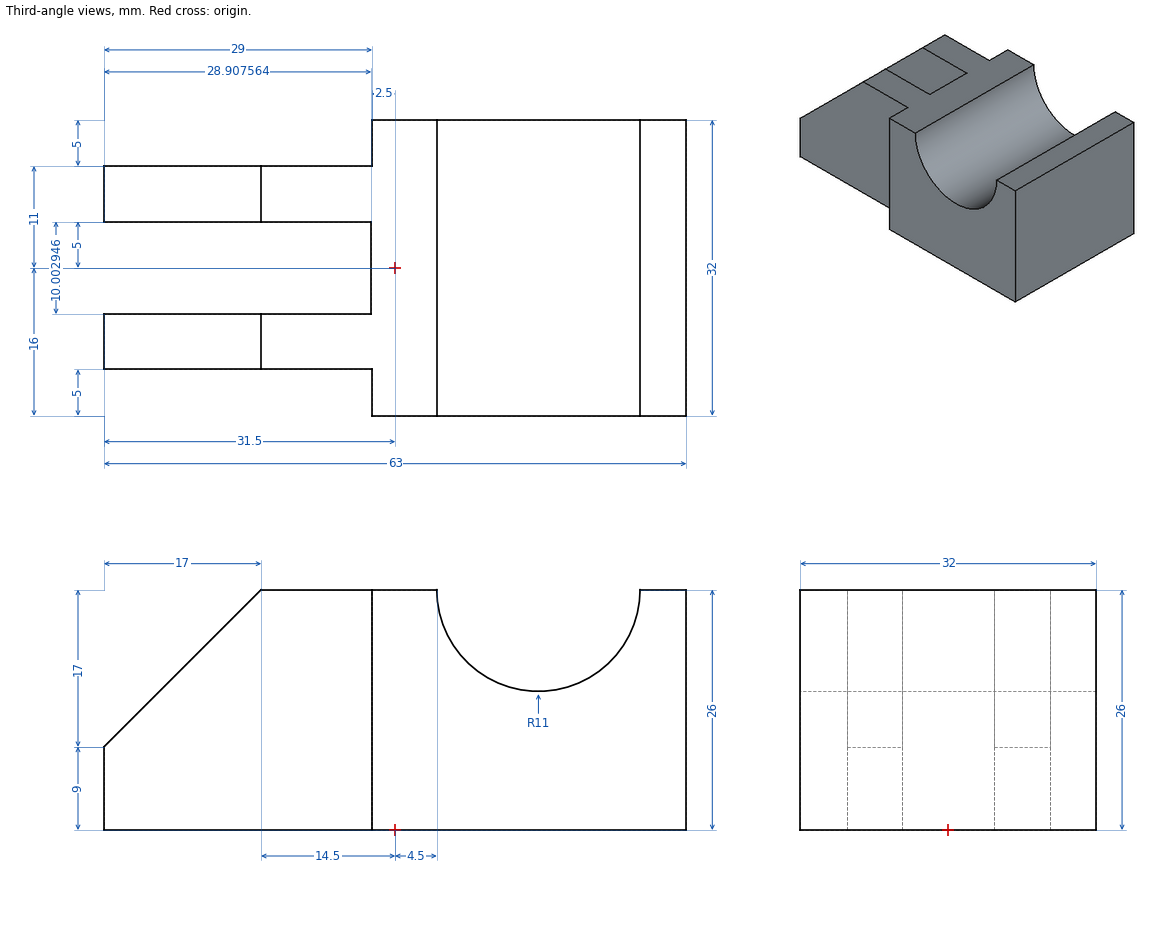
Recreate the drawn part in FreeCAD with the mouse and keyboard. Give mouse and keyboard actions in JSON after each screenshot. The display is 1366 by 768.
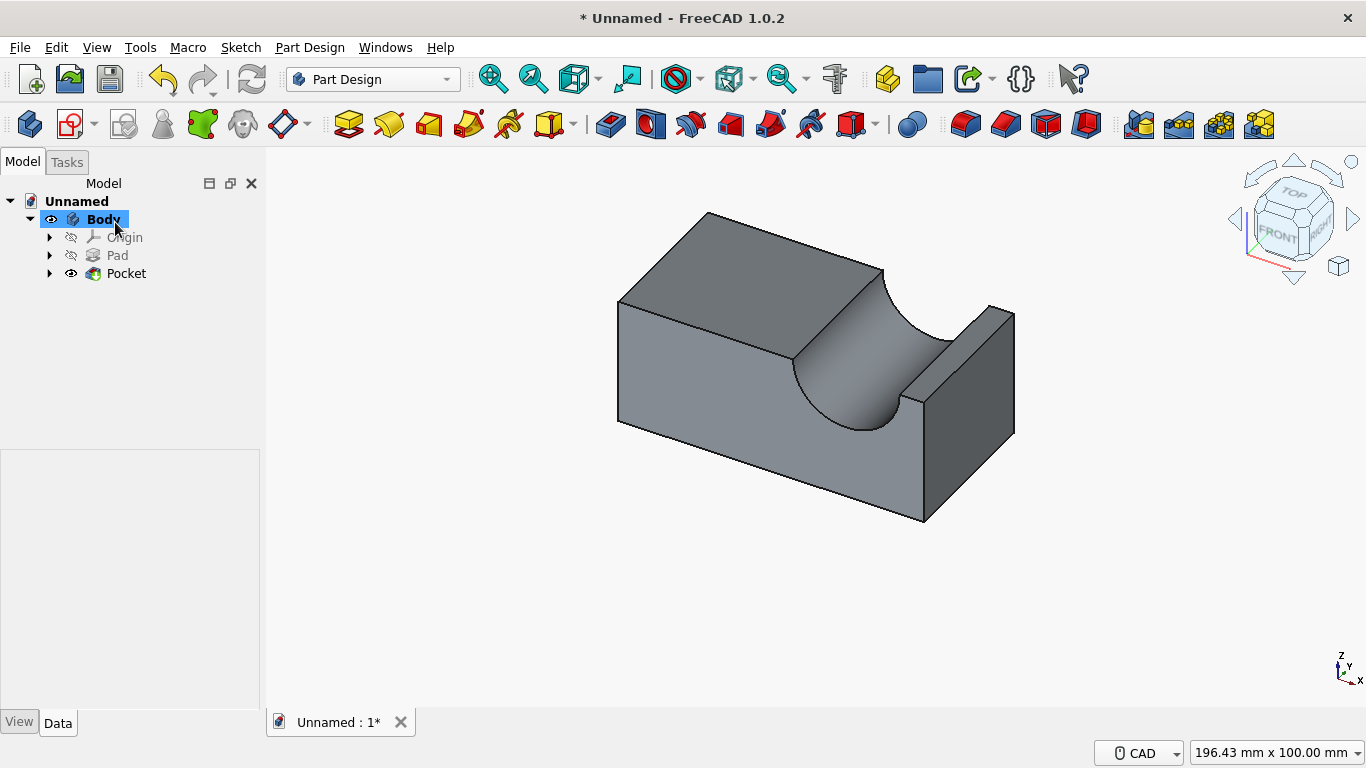
{"action": "left_click", "coordinate": [728, 396]}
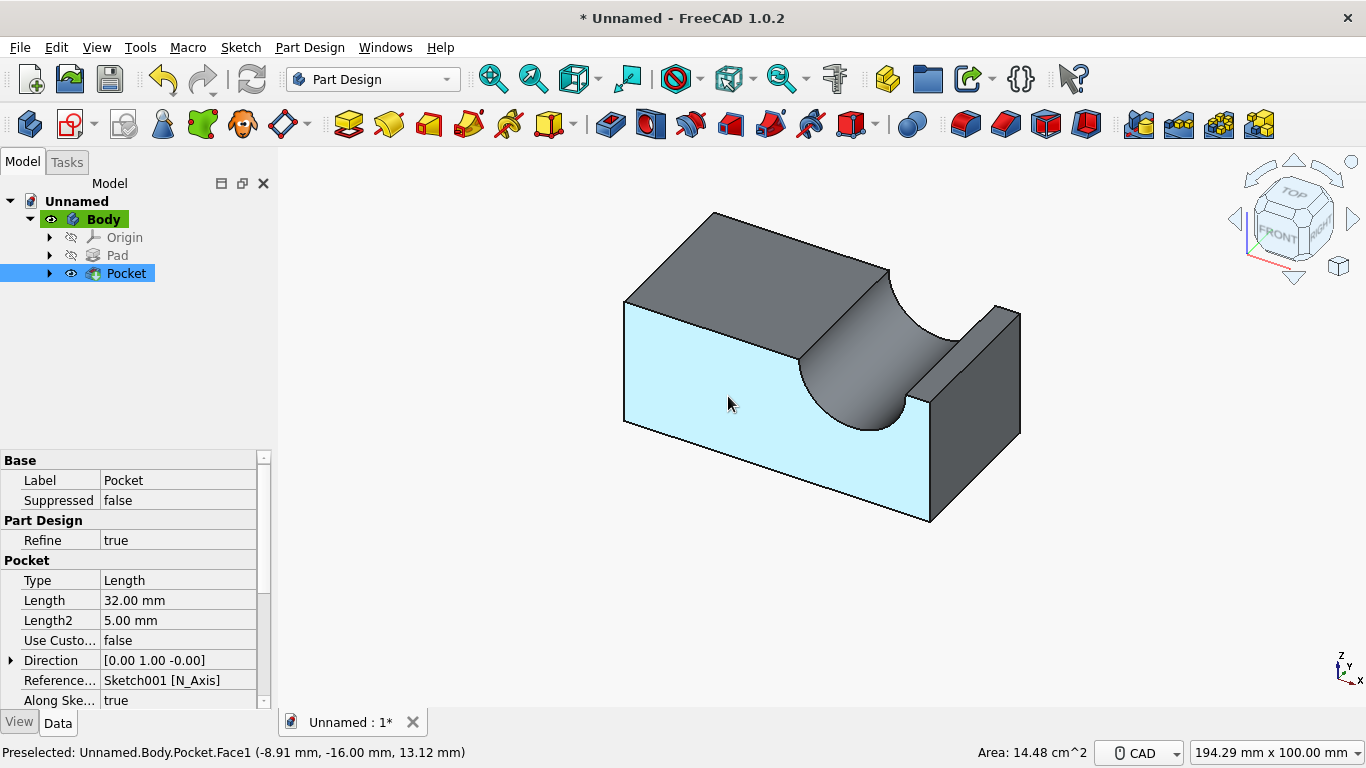
{"action": "left_click", "coordinate": [70, 124]}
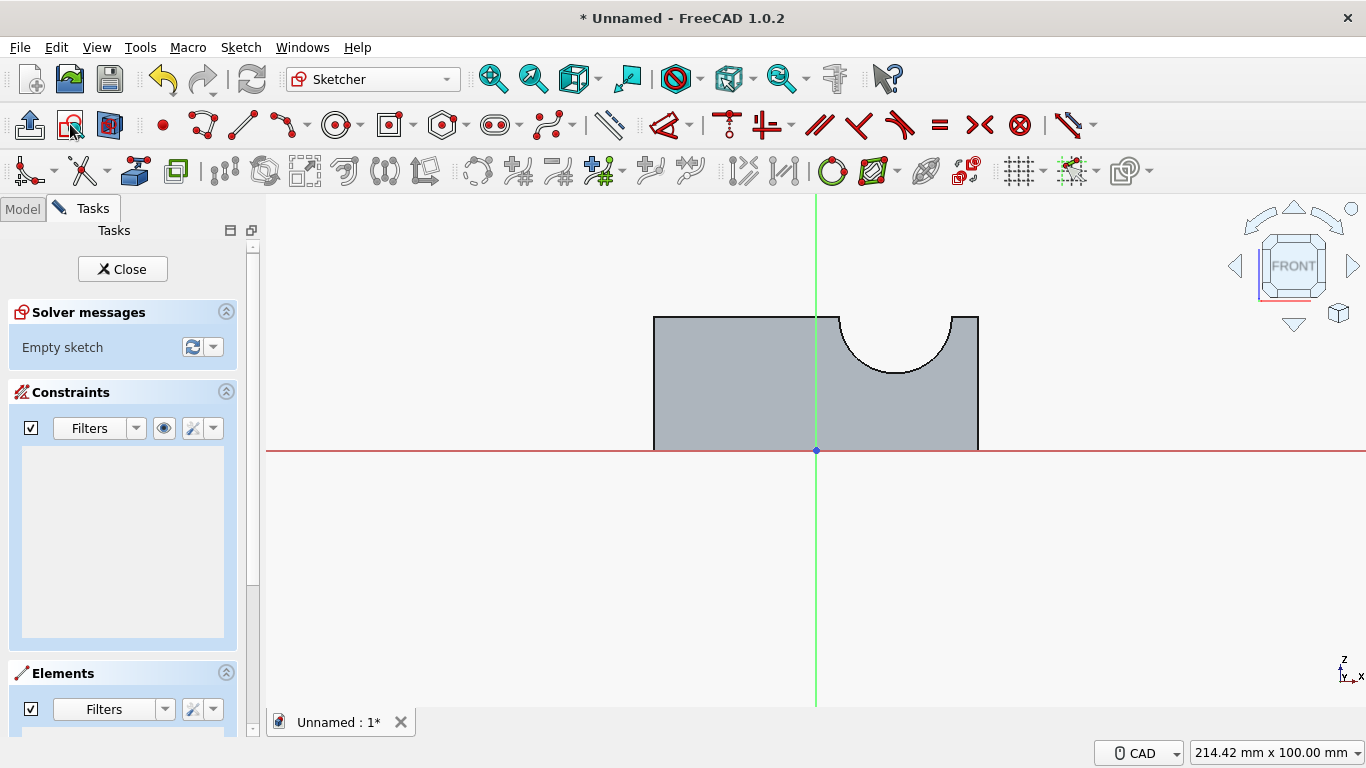
{"action": "scroll", "coordinate": [725, 329], "scroll_direction": "up", "scroll_amount": 4}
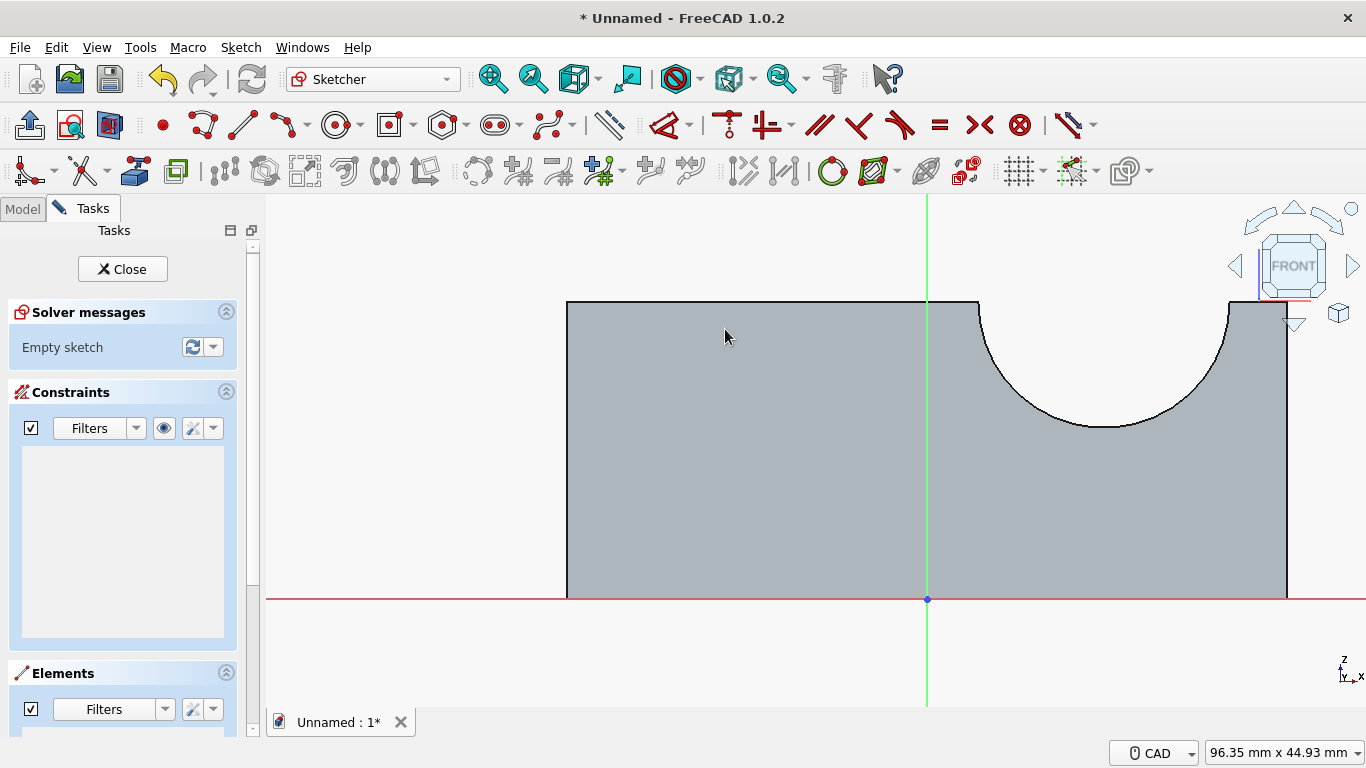
{"action": "left_click", "coordinate": [204, 126]}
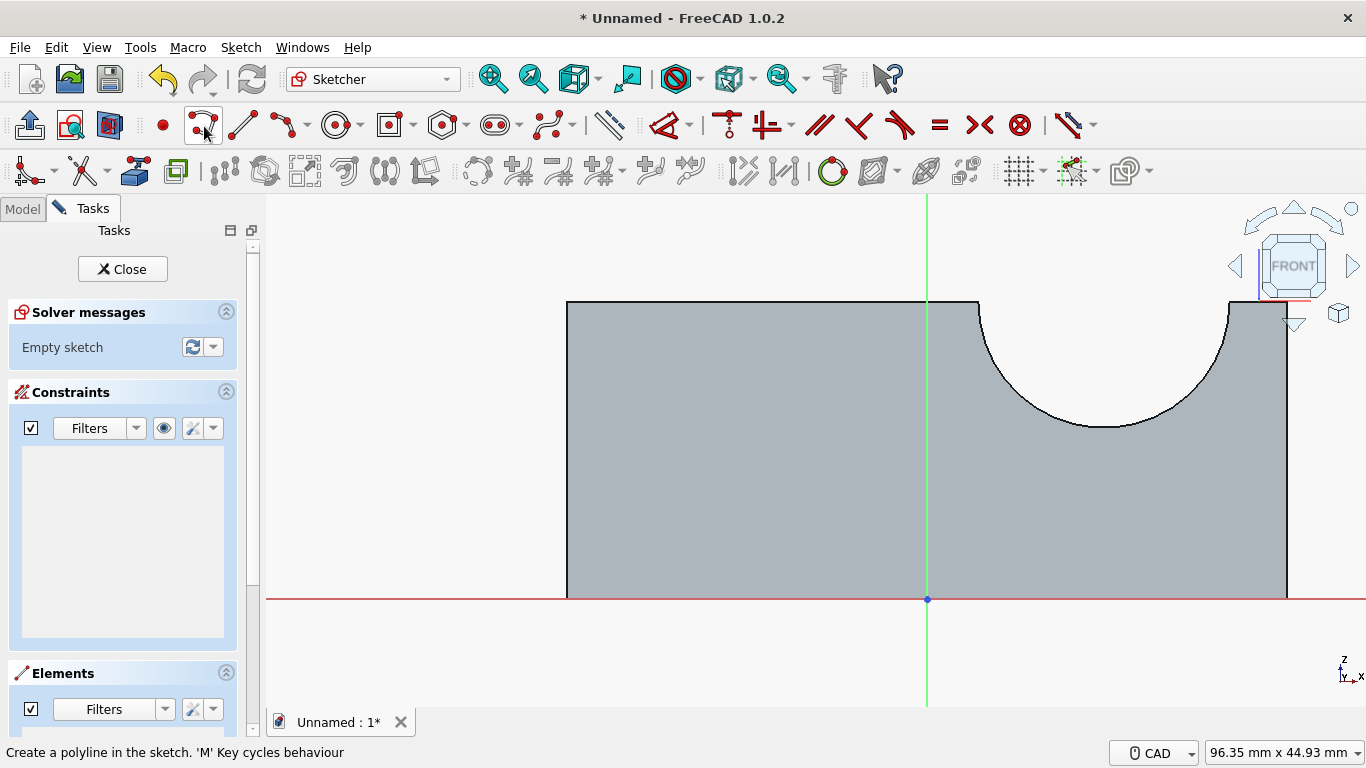
{"action": "left_click", "coordinate": [761, 302]}
{"action": "left_click", "coordinate": [567, 302]}
{"action": "left_click", "coordinate": [567, 496]}
{"action": "left_click", "coordinate": [761, 303]}
{"action": "key", "text": "Escape"}
{"action": "key", "text": "Escape"}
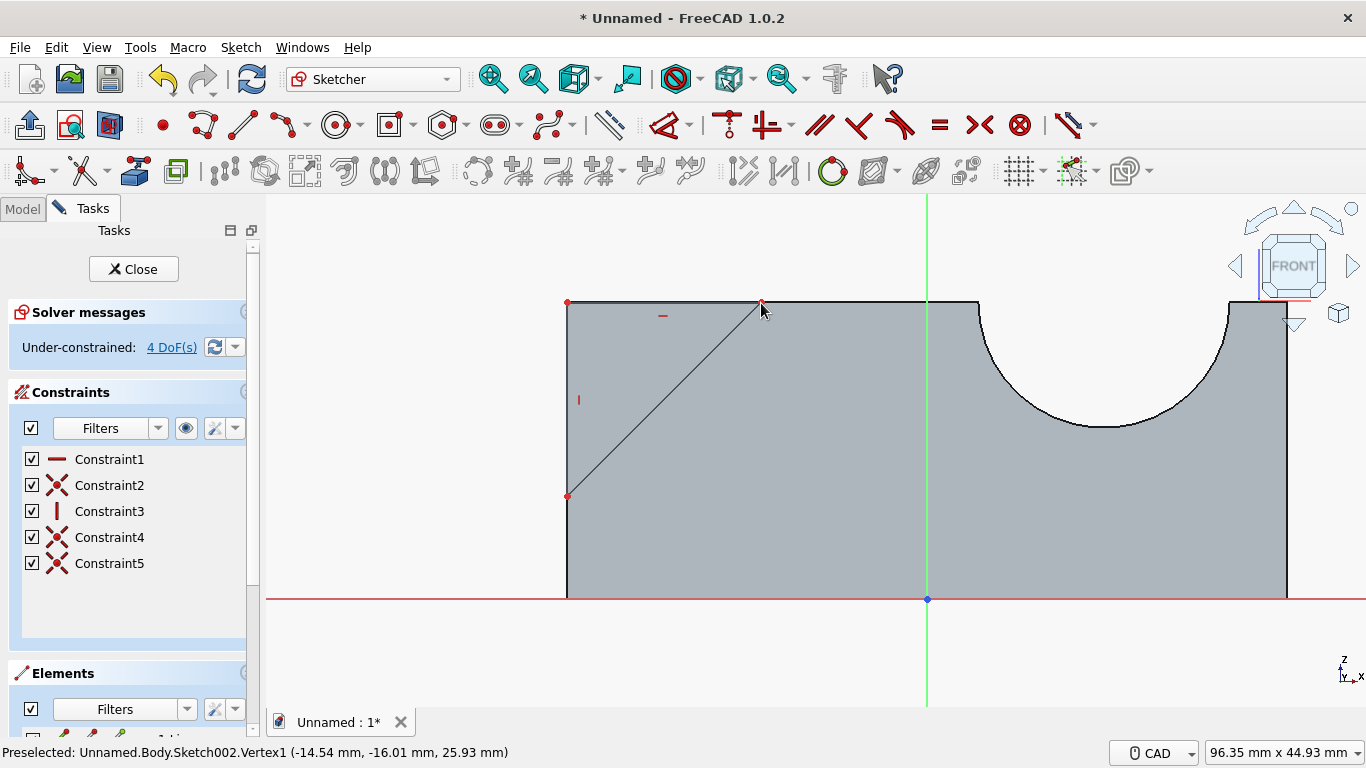
{"action": "left_click", "coordinate": [664, 126]}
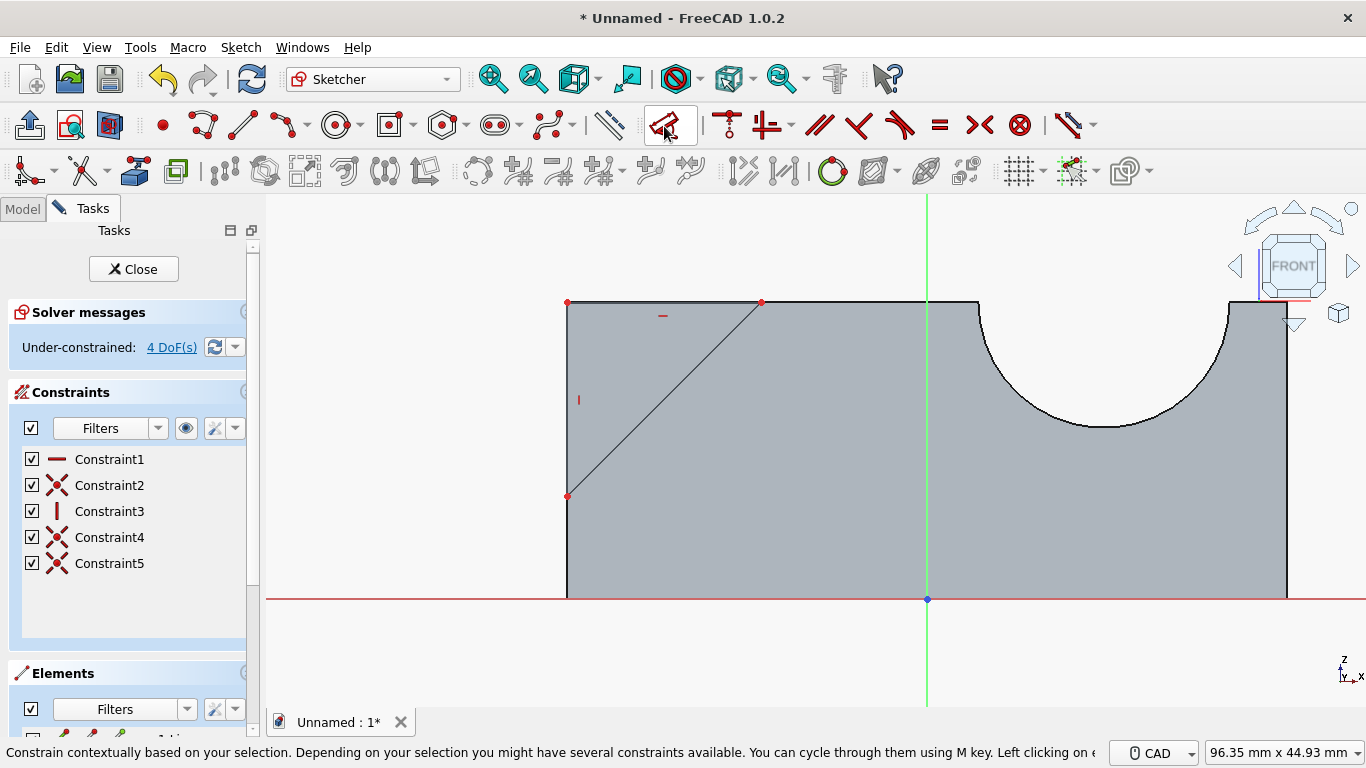
{"action": "left_click", "coordinate": [703, 303]}
{"action": "left_click", "coordinate": [664, 269]}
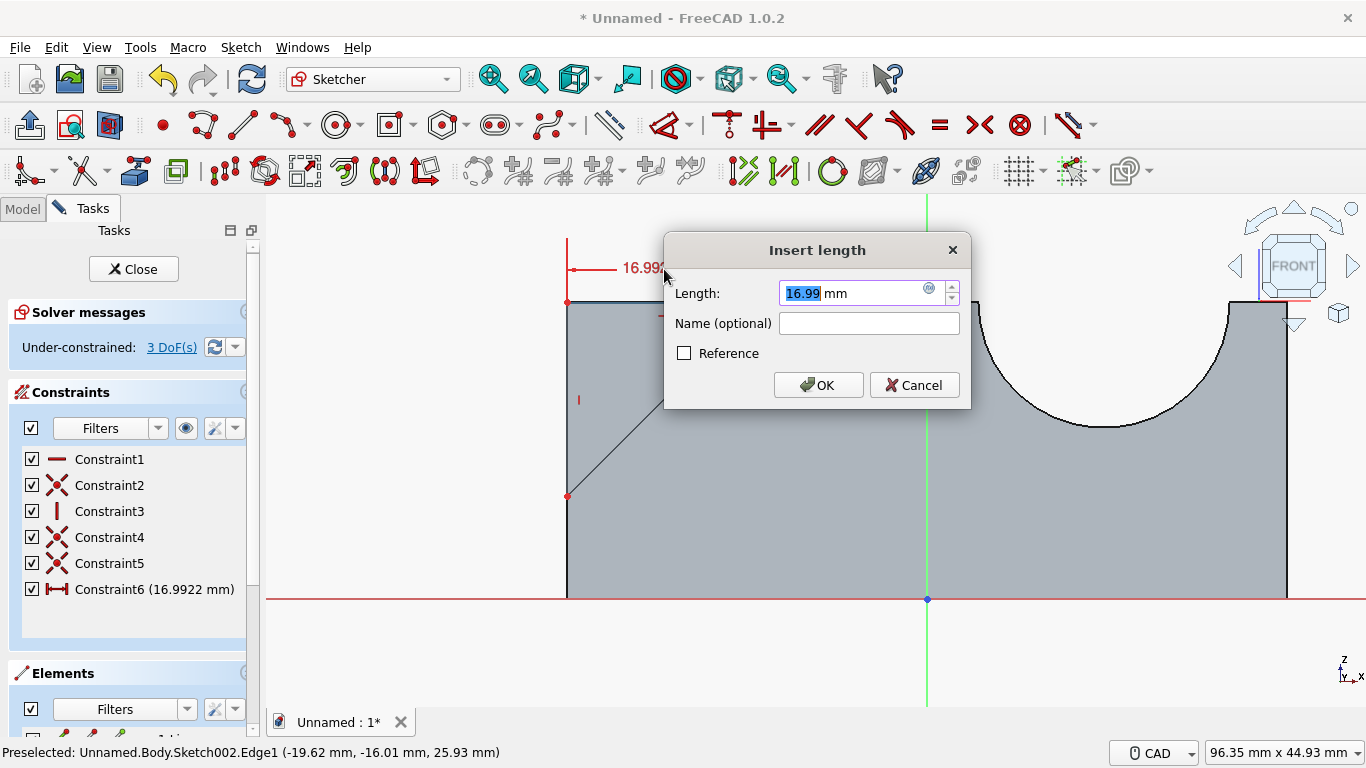
{"action": "type", "text": "17"}
{"action": "key", "text": "Return"}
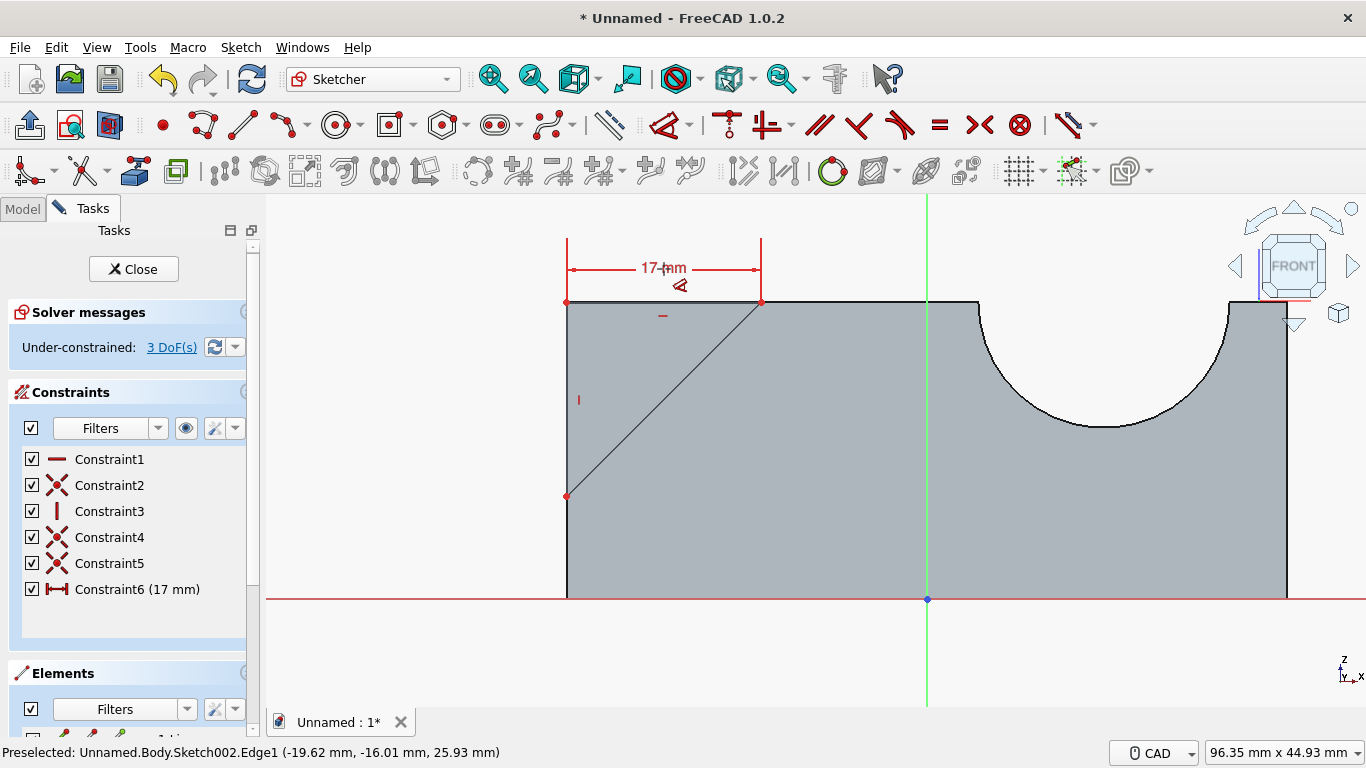
{"action": "left_click", "coordinate": [567, 361]}
{"action": "left_click", "coordinate": [533, 400]}